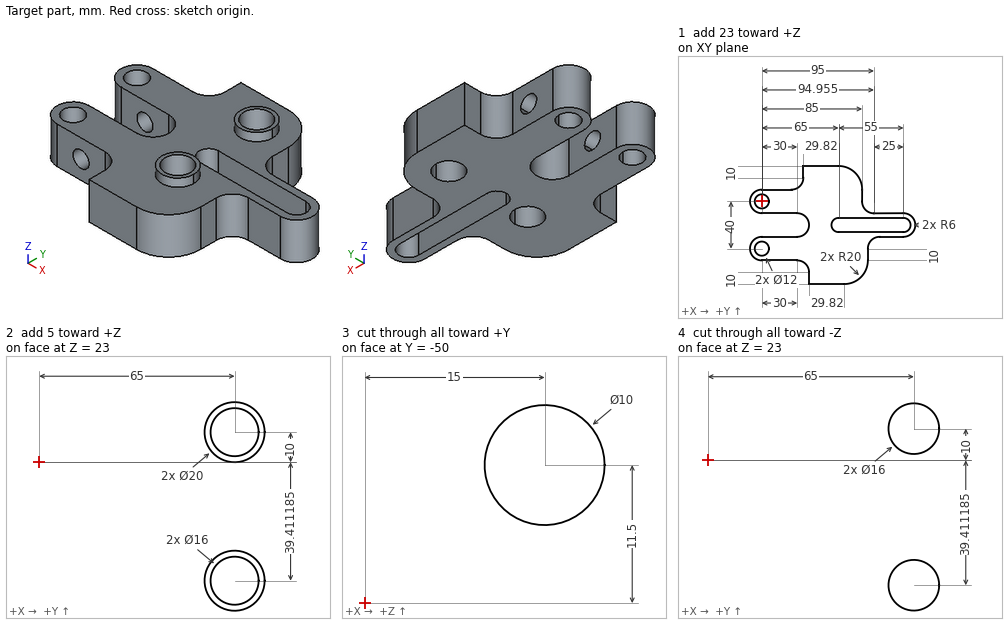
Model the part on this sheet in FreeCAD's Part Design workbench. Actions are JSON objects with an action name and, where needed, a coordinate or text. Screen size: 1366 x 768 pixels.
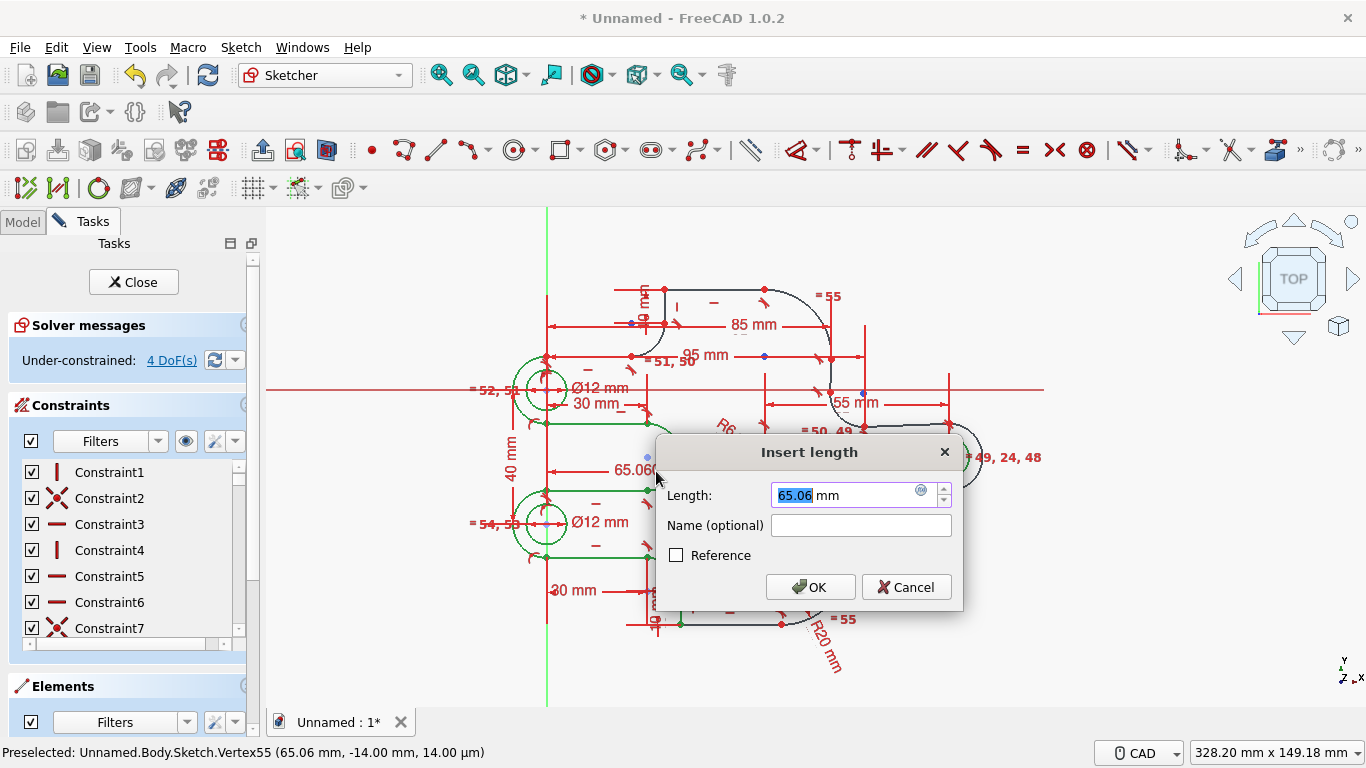
{"action": "type", "text": "65"}
{"action": "key", "text": "Return"}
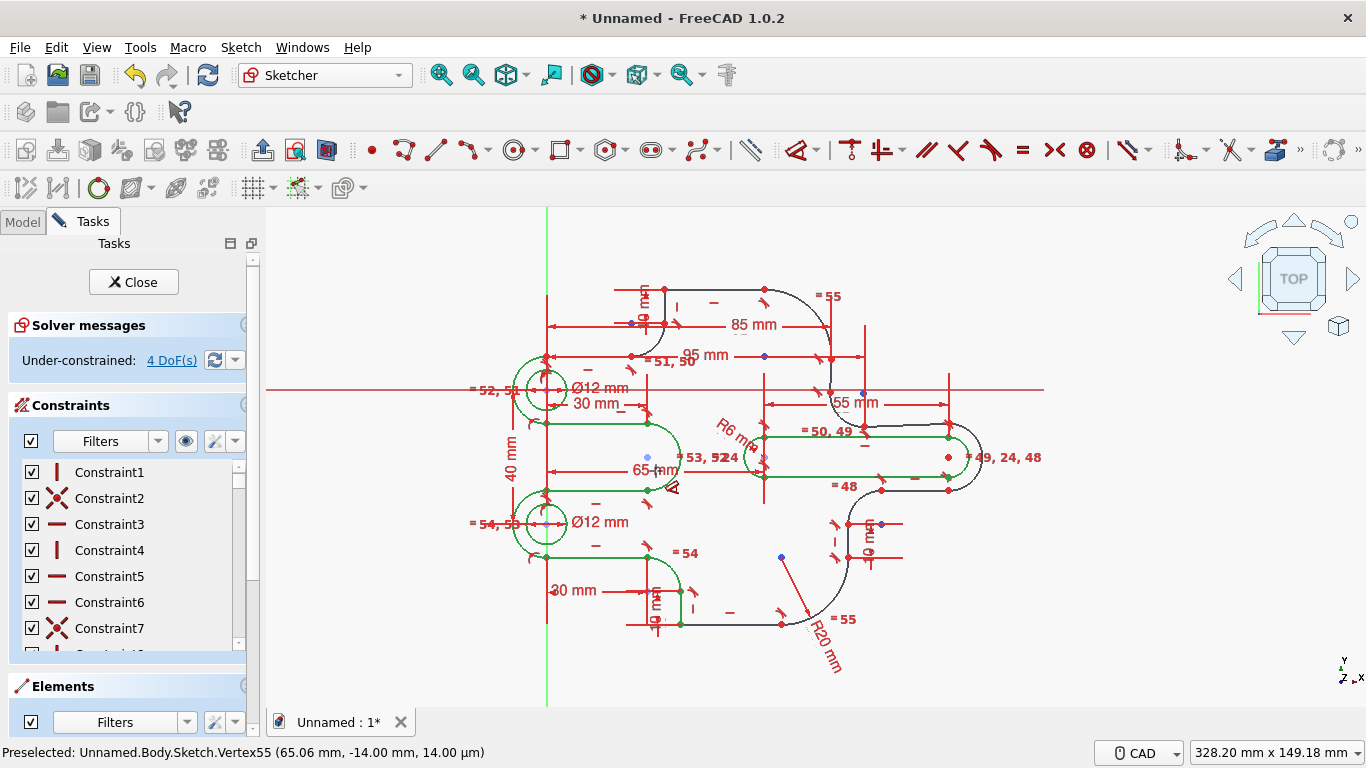
{"action": "left_click", "coordinate": [924, 425]}
{"action": "left_click", "coordinate": [907, 461]}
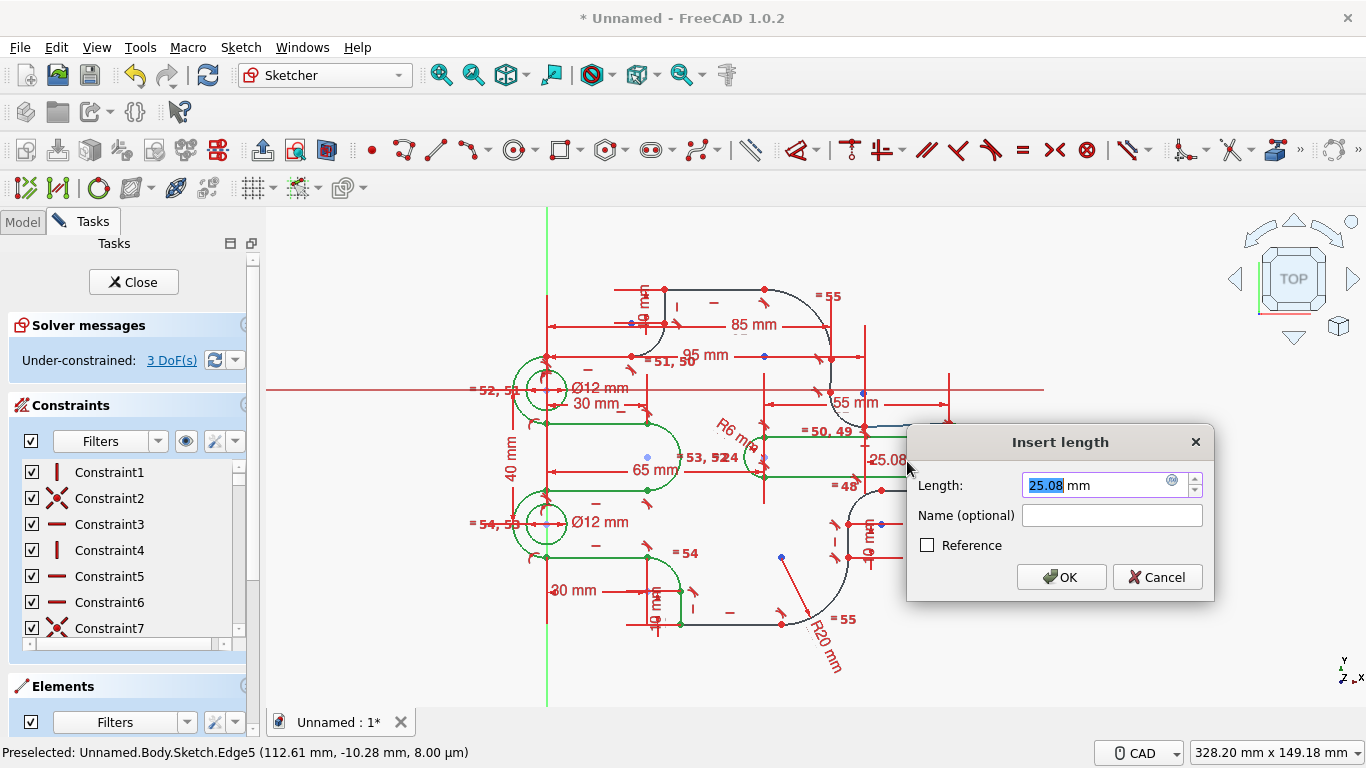
{"action": "type", "text": "25"}
{"action": "key", "text": "Return"}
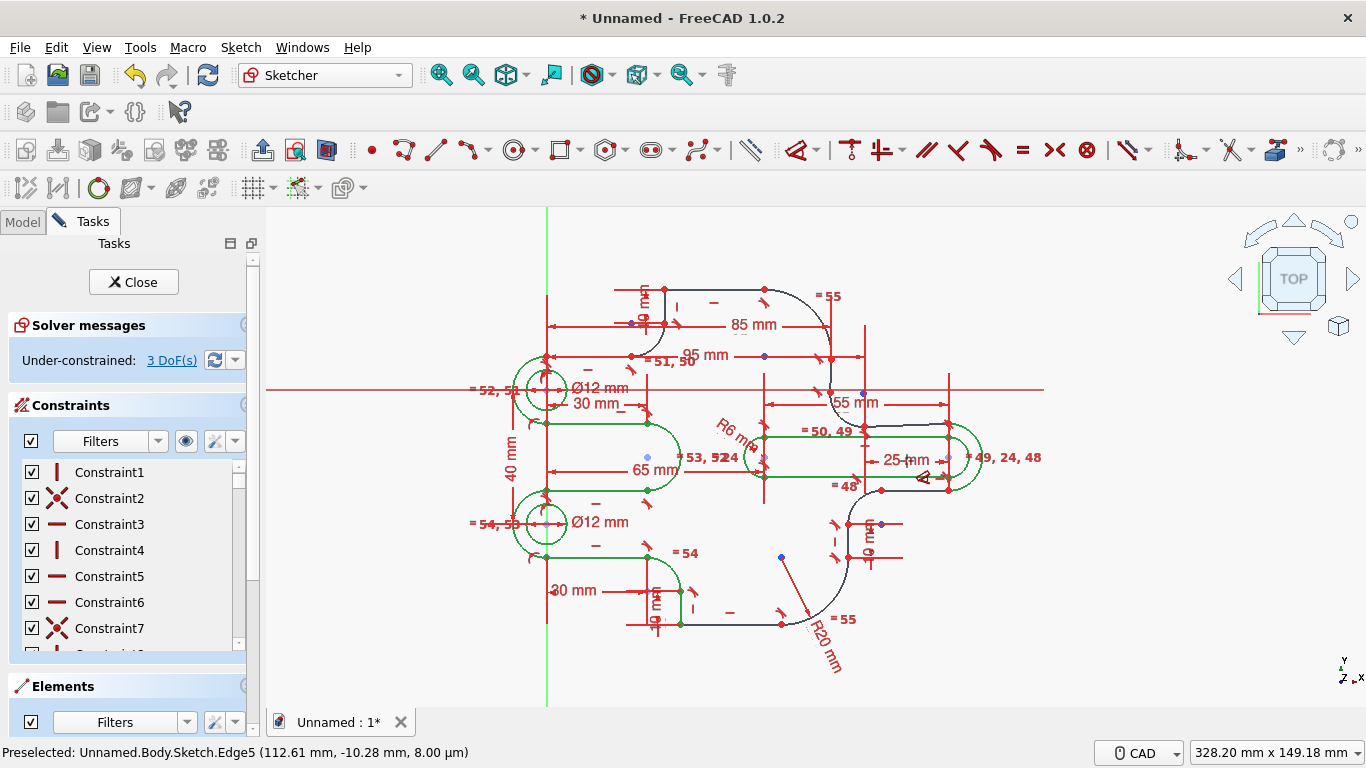
{"action": "left_click", "coordinate": [711, 625]}
{"action": "left_click", "coordinate": [731, 659]}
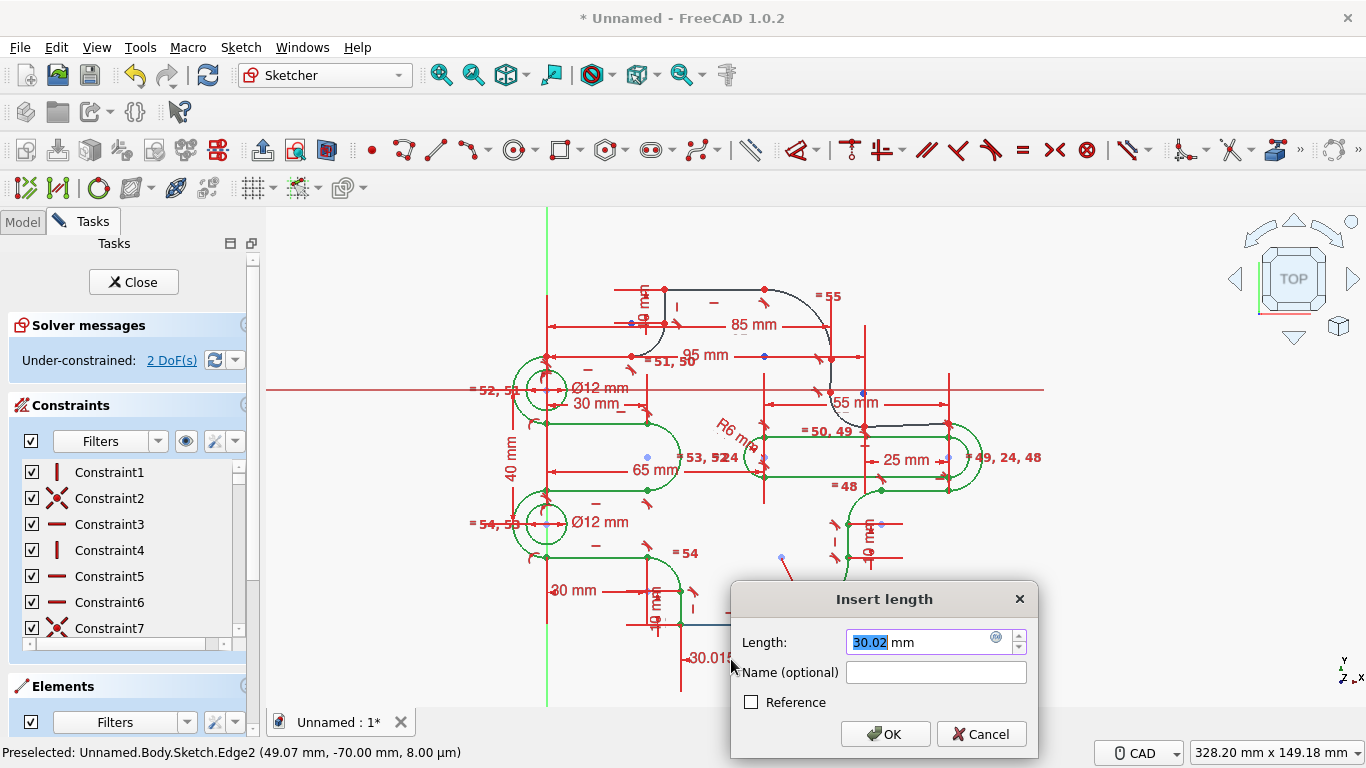
{"action": "type", "text": "29.82"}
{"action": "key", "text": "Return"}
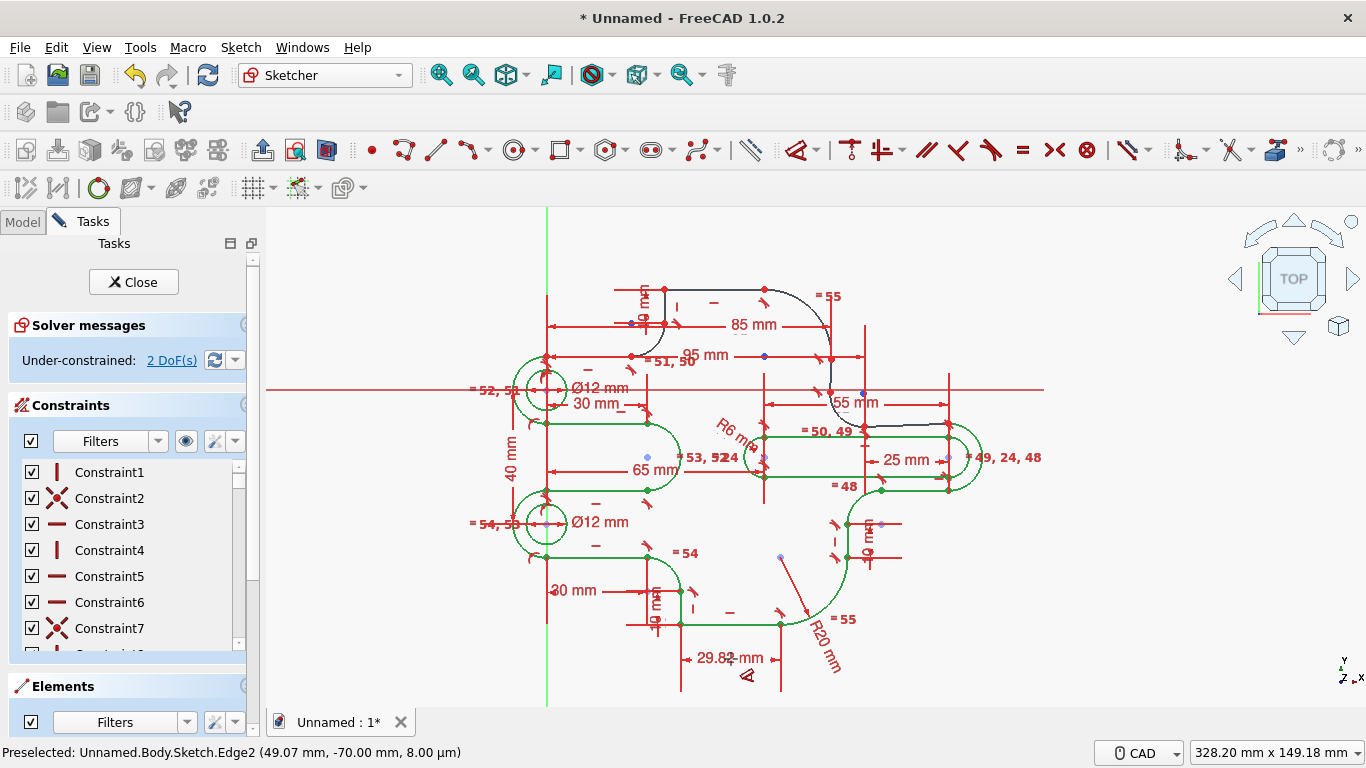
{"action": "left_click", "coordinate": [734, 290]}
{"action": "left_click", "coordinate": [715, 256]}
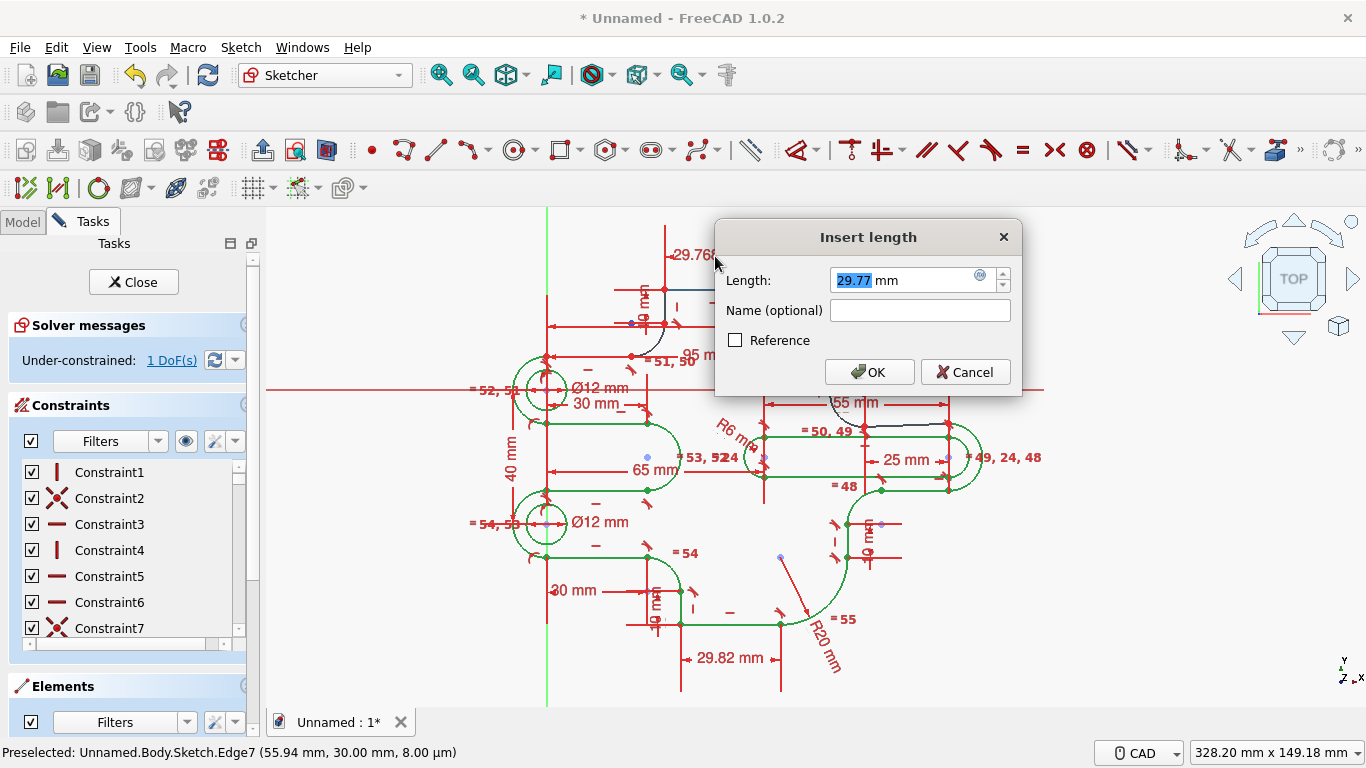
{"action": "type", "text": "29.82"}
{"action": "key", "text": "Return"}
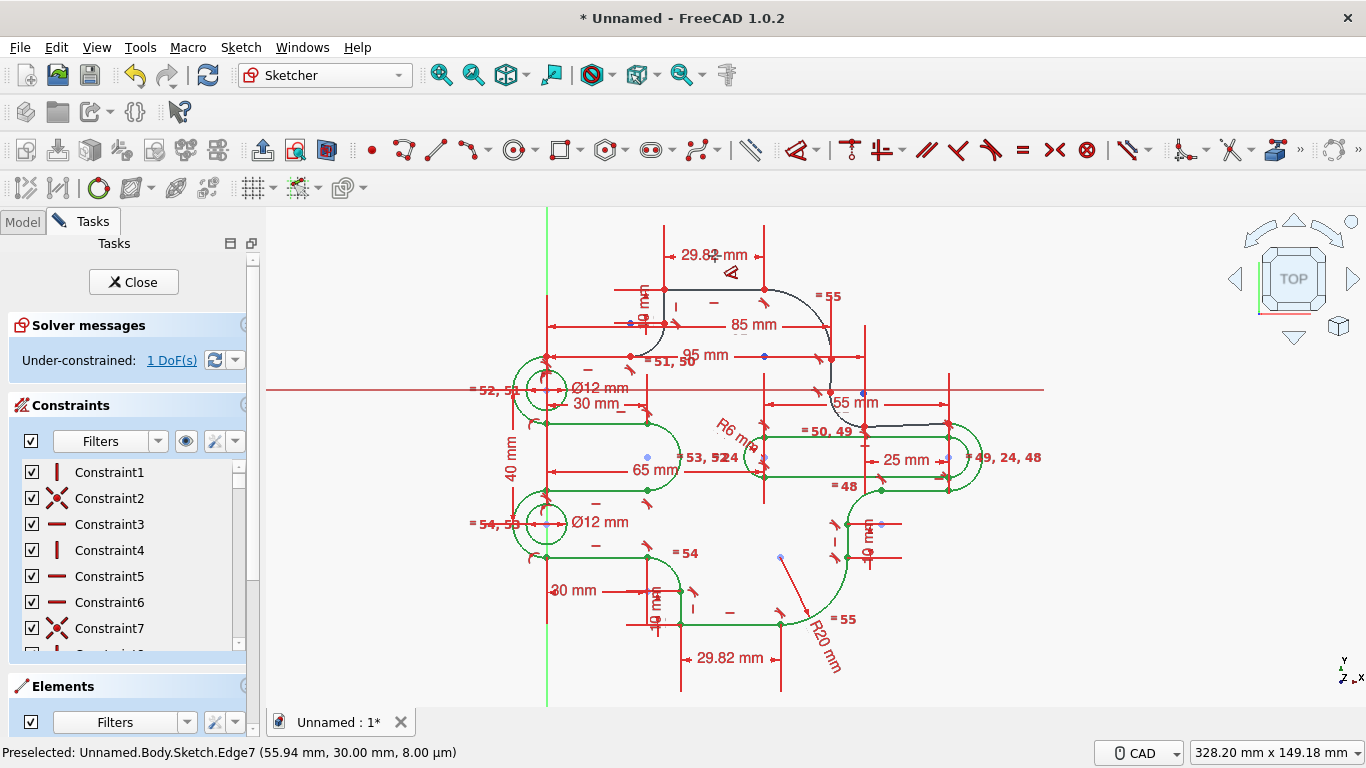
{"action": "left_click", "coordinate": [864, 393]}
{"action": "left_click", "coordinate": [778, 356]}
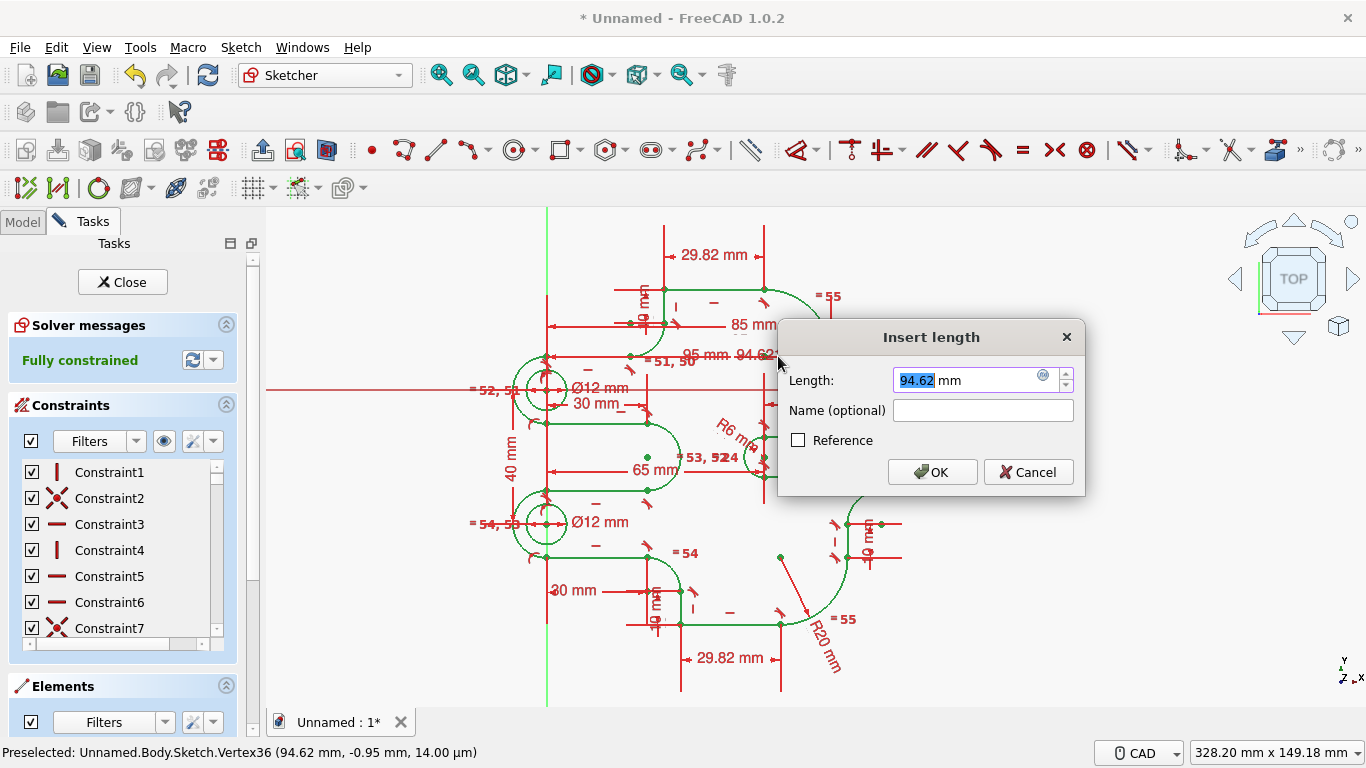
{"action": "type", "text": "94.955"}
{"action": "key", "text": "Return"}
{"action": "key", "text": "Escape"}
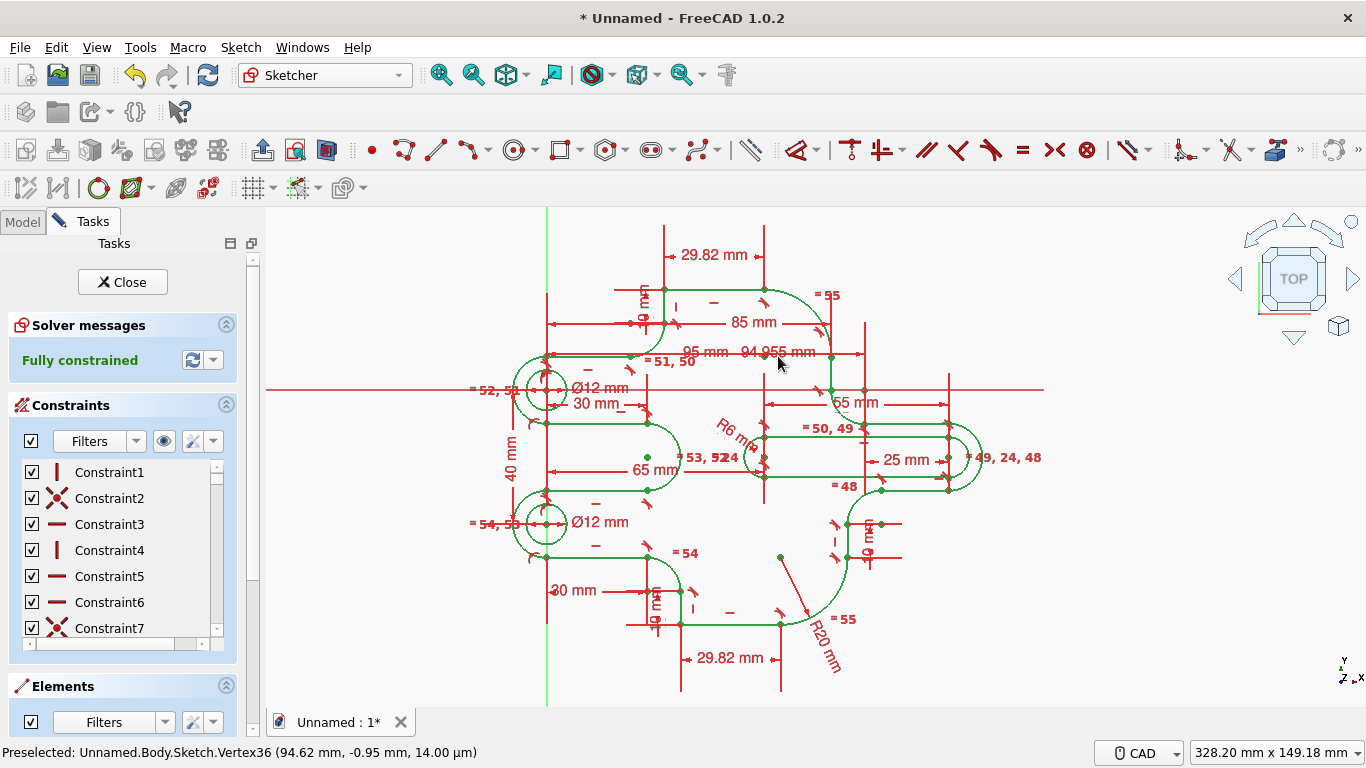
{"action": "left_click", "coordinate": [123, 282]}